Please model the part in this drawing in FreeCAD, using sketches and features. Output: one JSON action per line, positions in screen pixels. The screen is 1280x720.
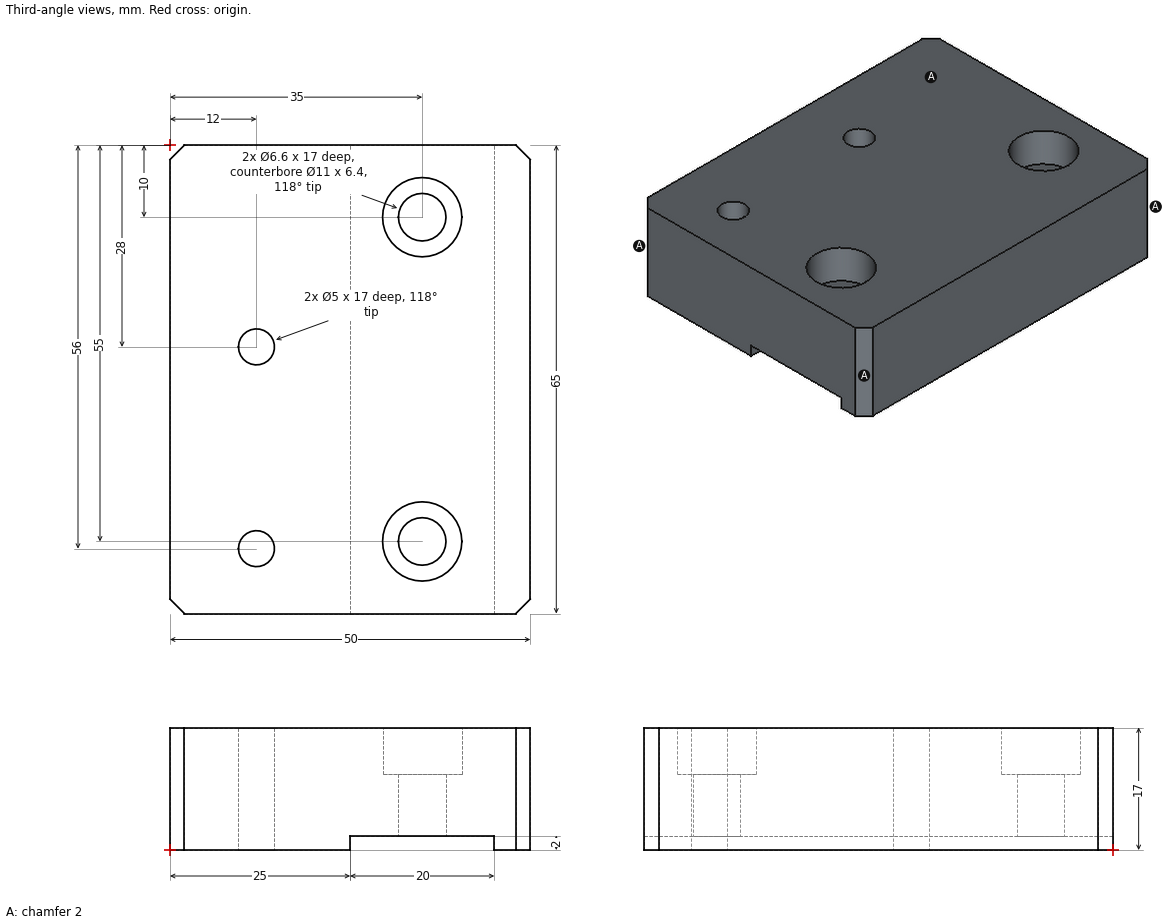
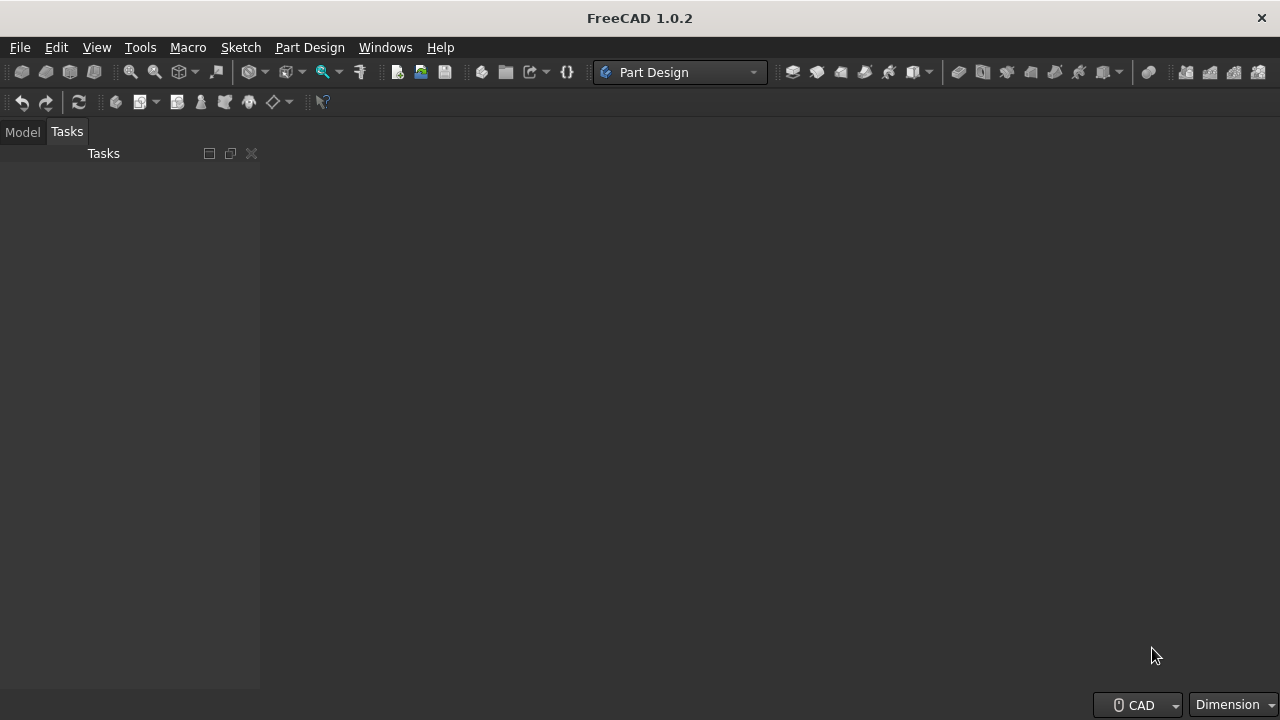
{"action": "left_click", "coordinate": [398, 72]}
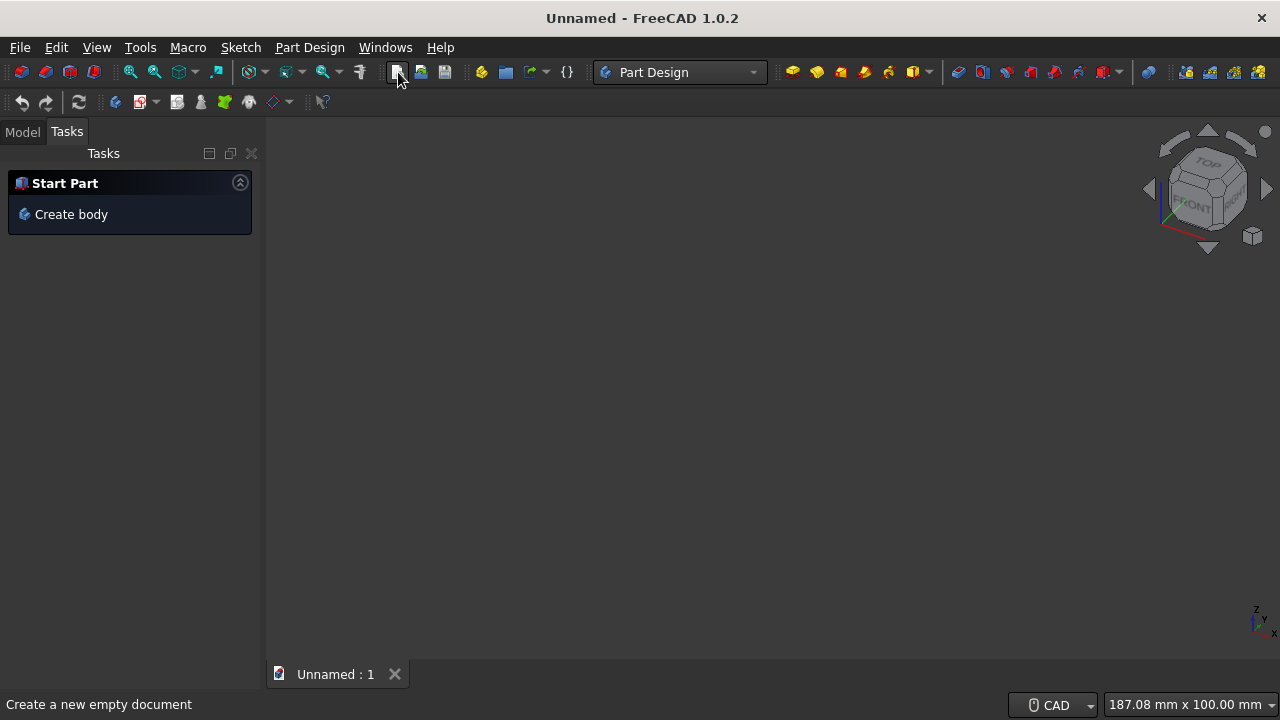
{"action": "left_click", "coordinate": [140, 102]}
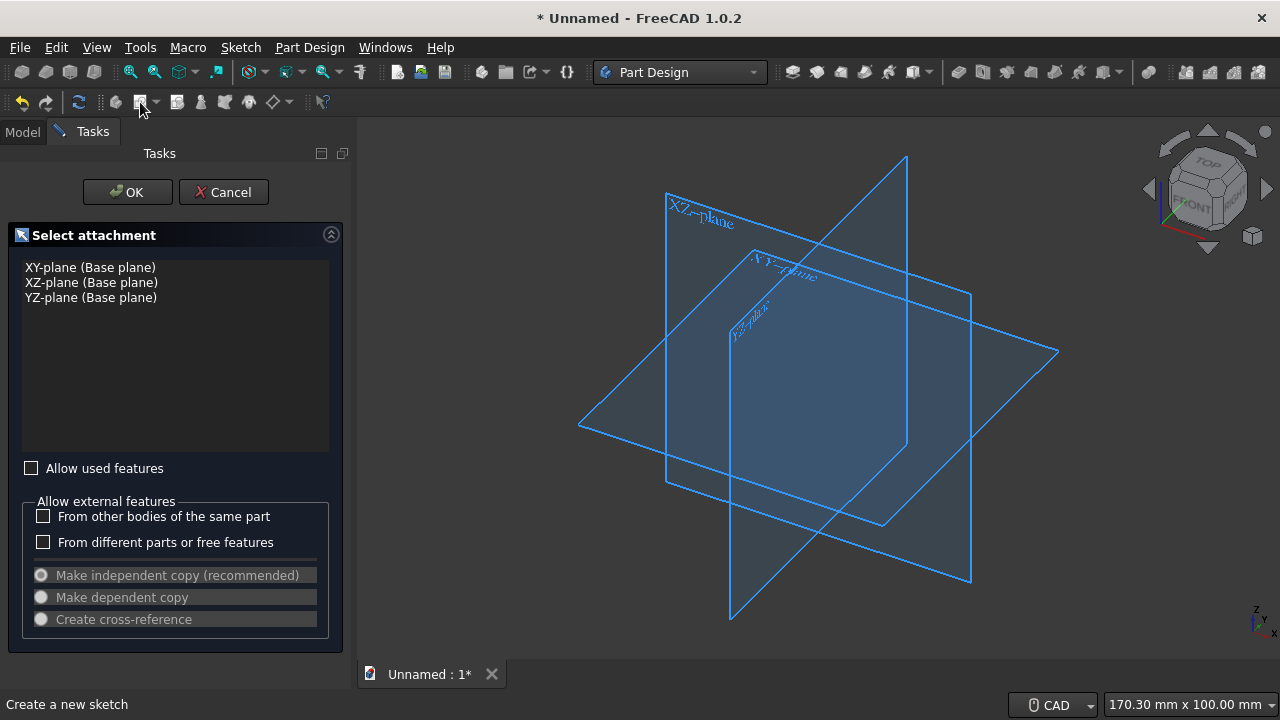
{"action": "left_click", "coordinate": [82, 268]}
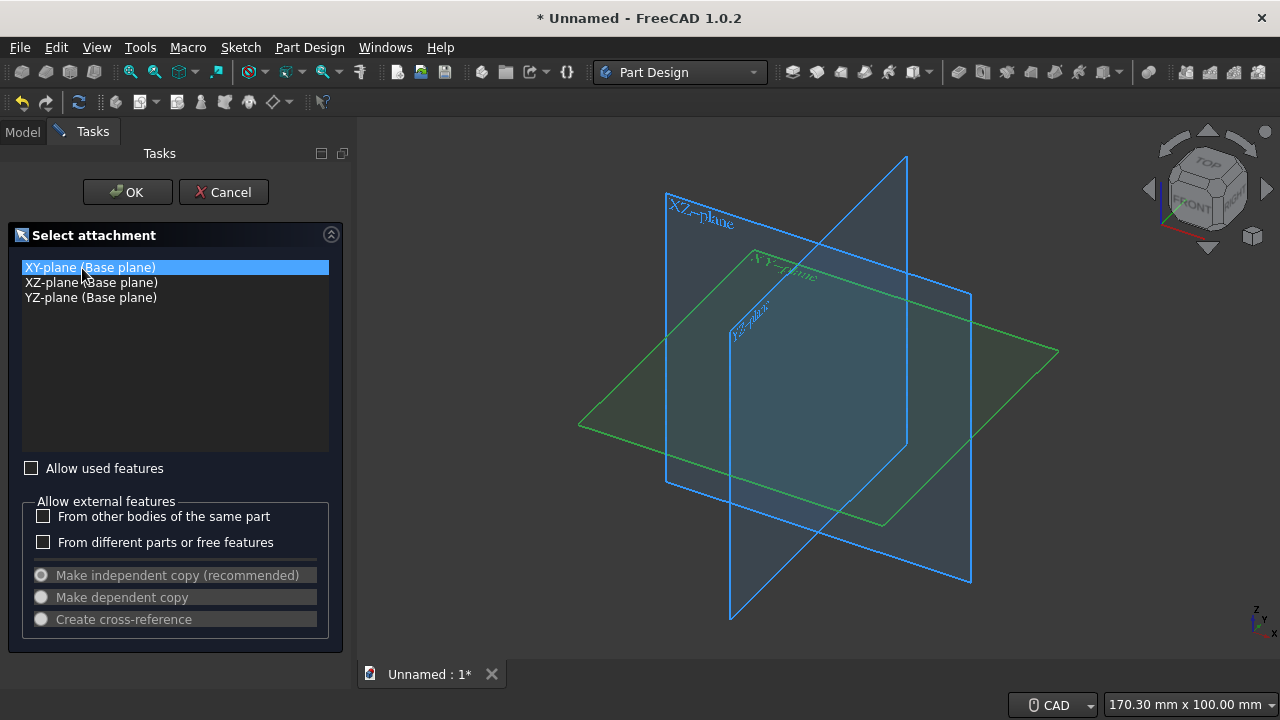
{"action": "left_click", "coordinate": [128, 192]}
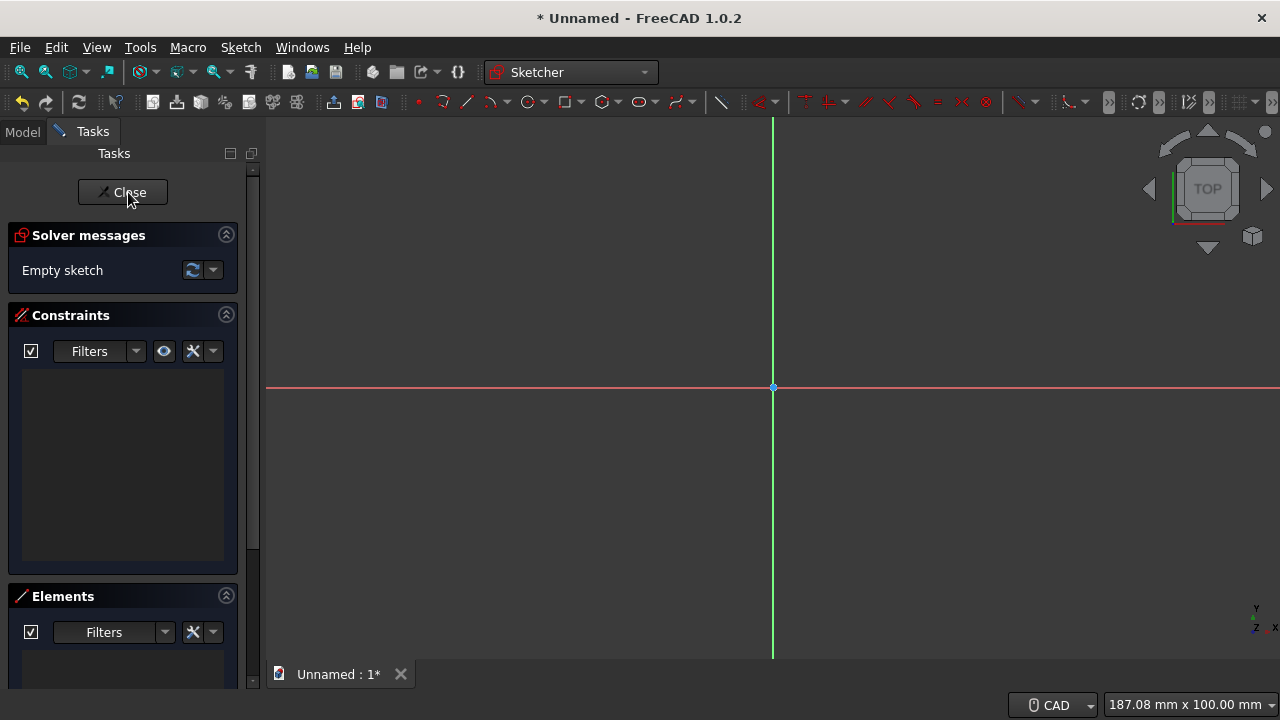
{"action": "scroll", "coordinate": [294, 145], "scroll_direction": "down", "scroll_amount": 2}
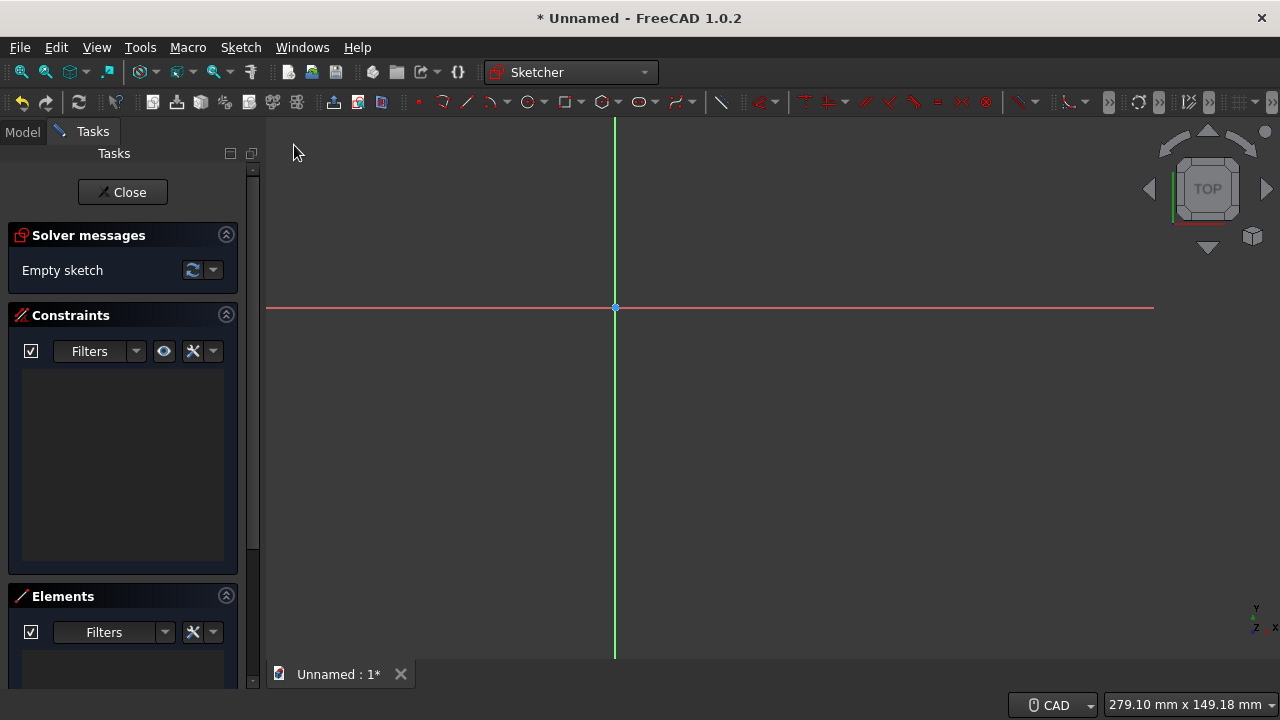
{"action": "scroll", "coordinate": [709, 503], "scroll_direction": "up", "scroll_amount": 2}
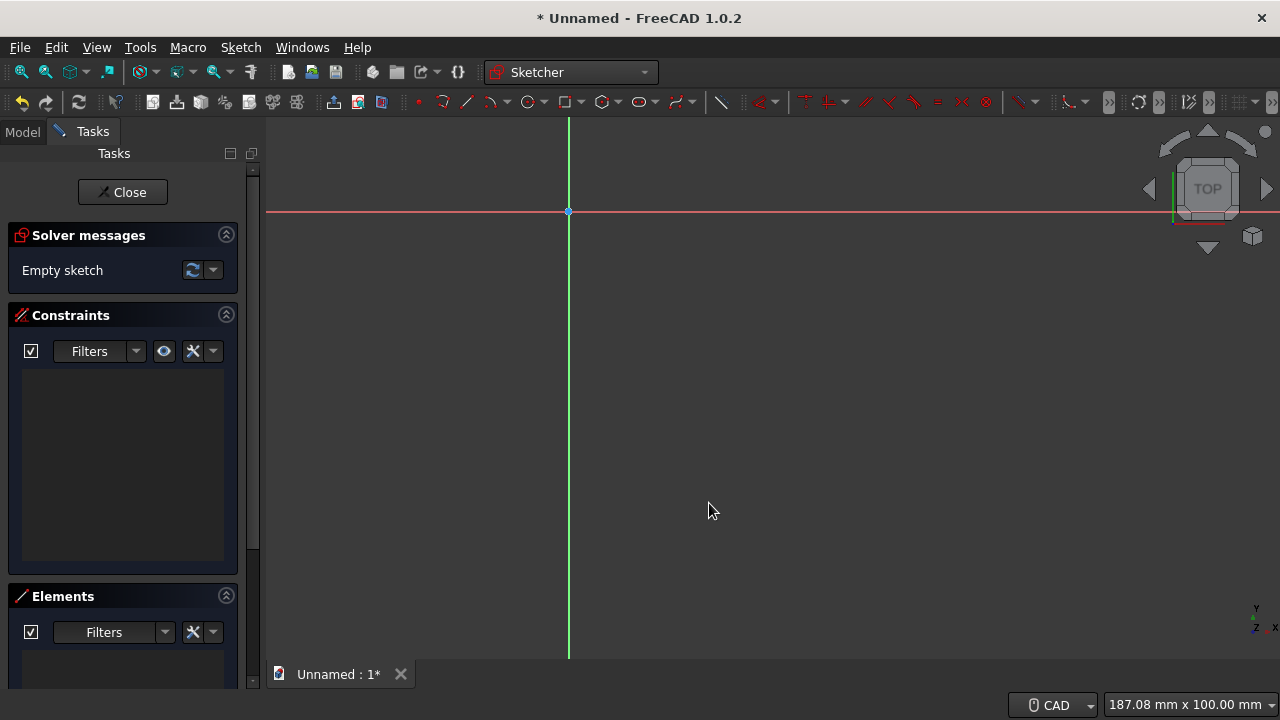
{"action": "left_click", "coordinate": [566, 102]}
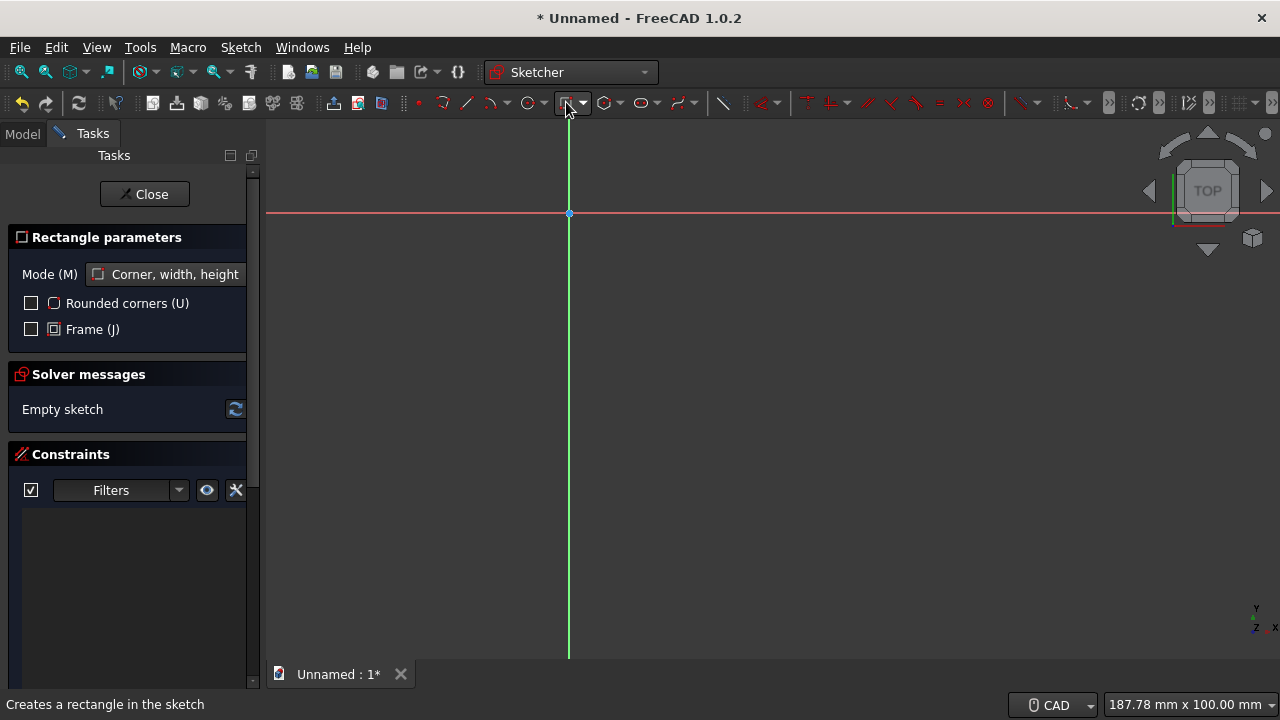
{"action": "left_click", "coordinate": [569, 213]}
{"action": "mouse_move", "coordinate": [839, 564]}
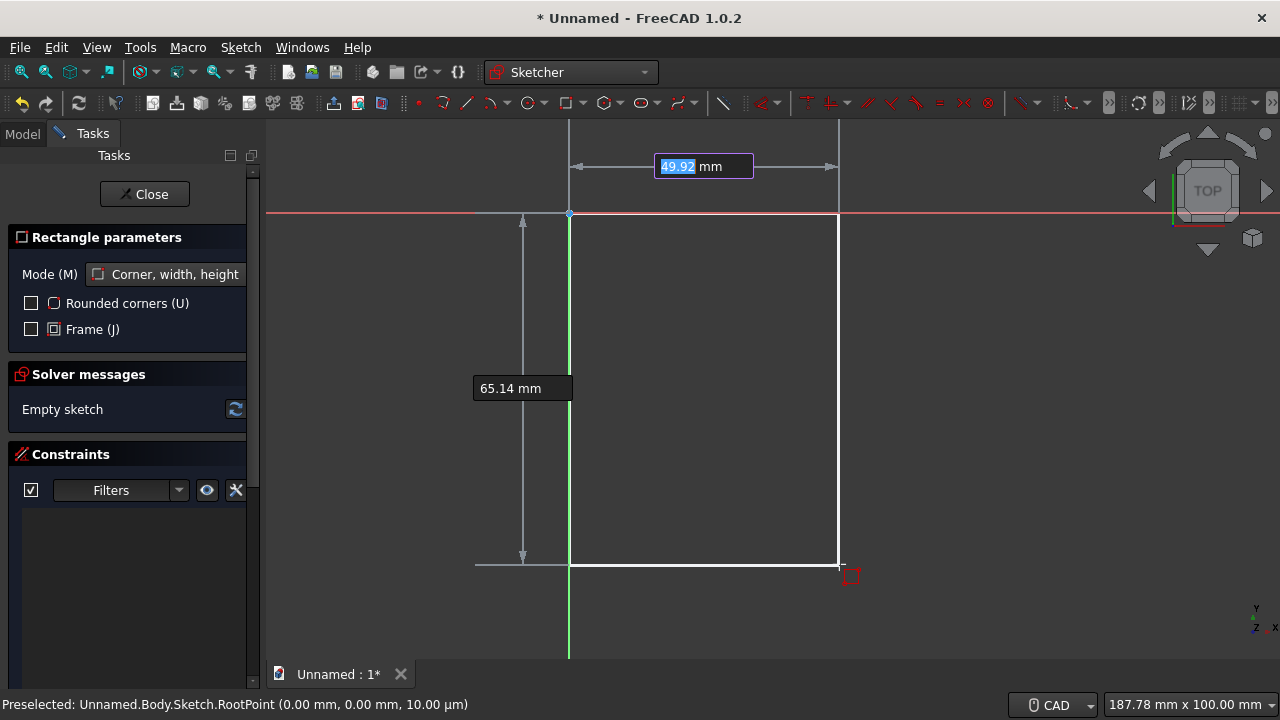
{"action": "type", "text": "50"}
{"action": "key", "text": "Tab"}
{"action": "type", "text": "65"}
{"action": "key", "text": "Return"}
{"action": "key", "text": "Escape"}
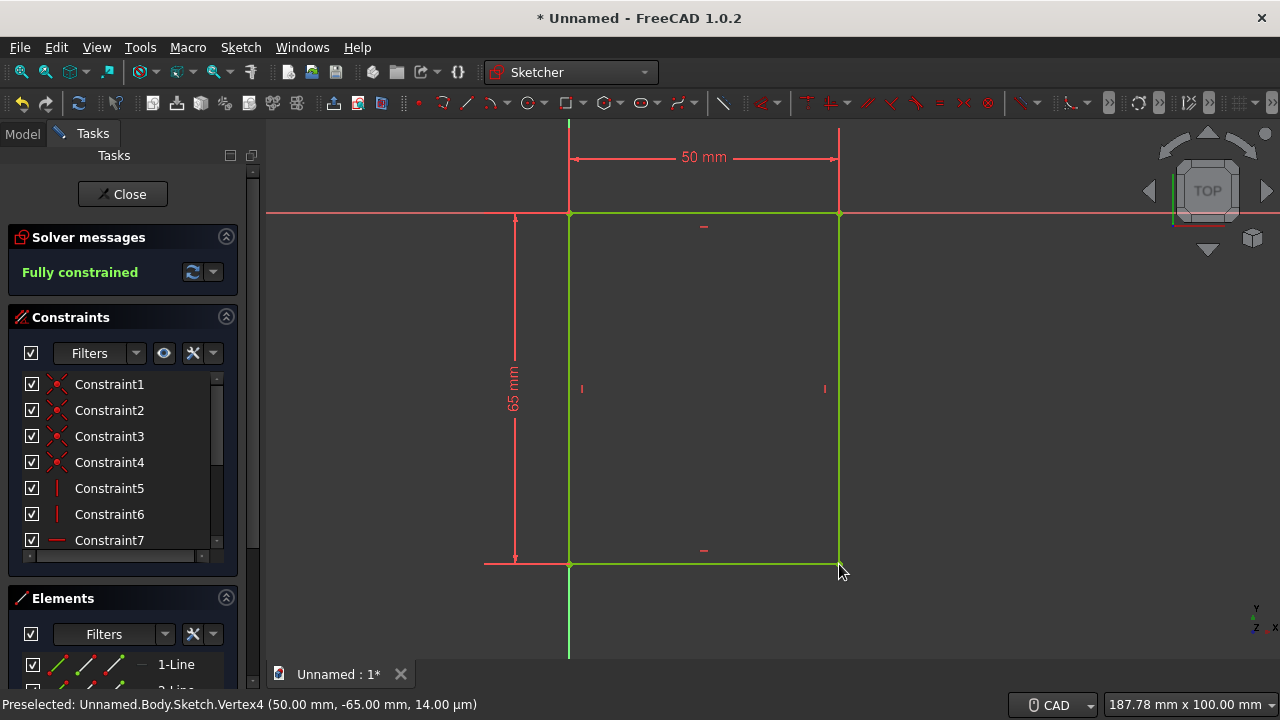
{"action": "left_click", "coordinate": [123, 194]}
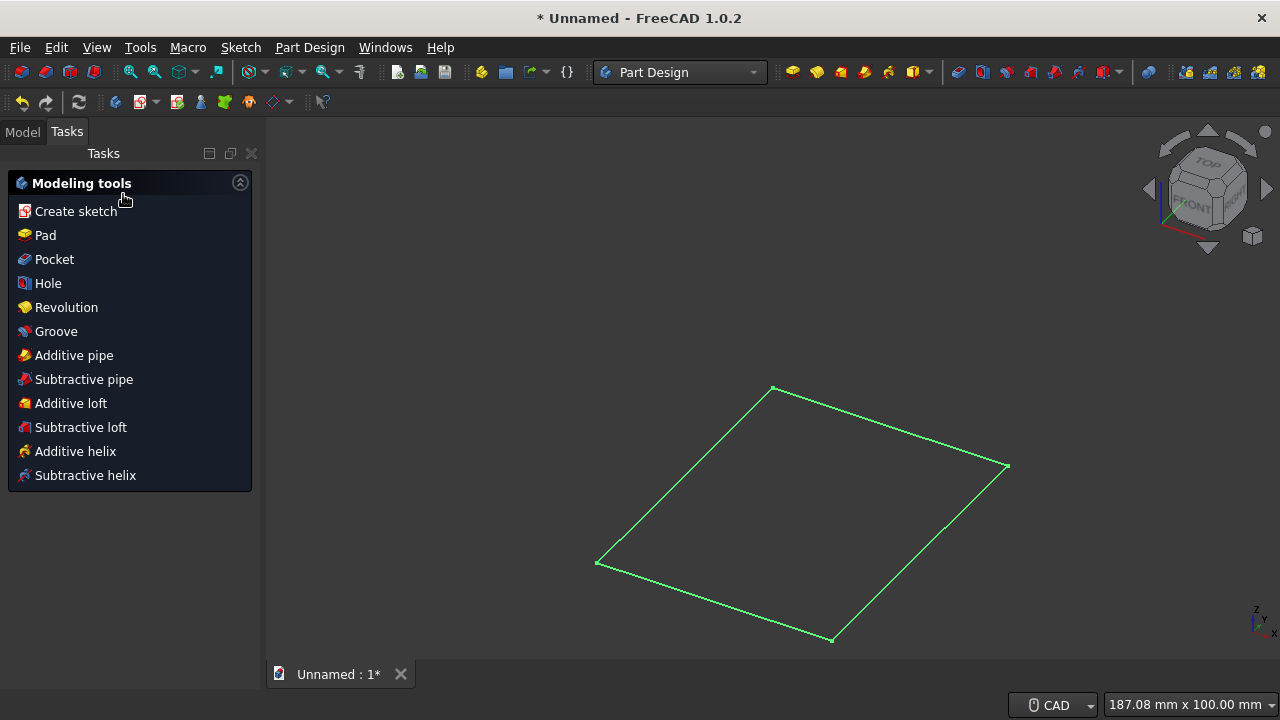
{"action": "left_click", "coordinate": [794, 72]}